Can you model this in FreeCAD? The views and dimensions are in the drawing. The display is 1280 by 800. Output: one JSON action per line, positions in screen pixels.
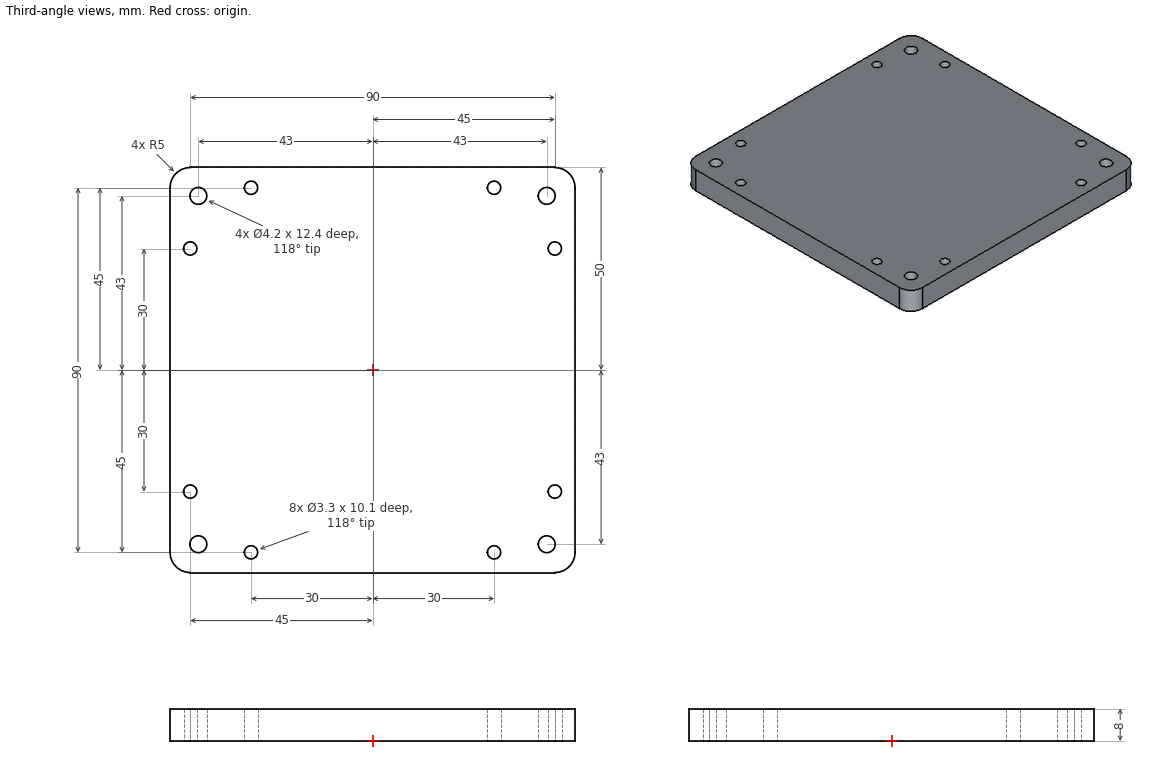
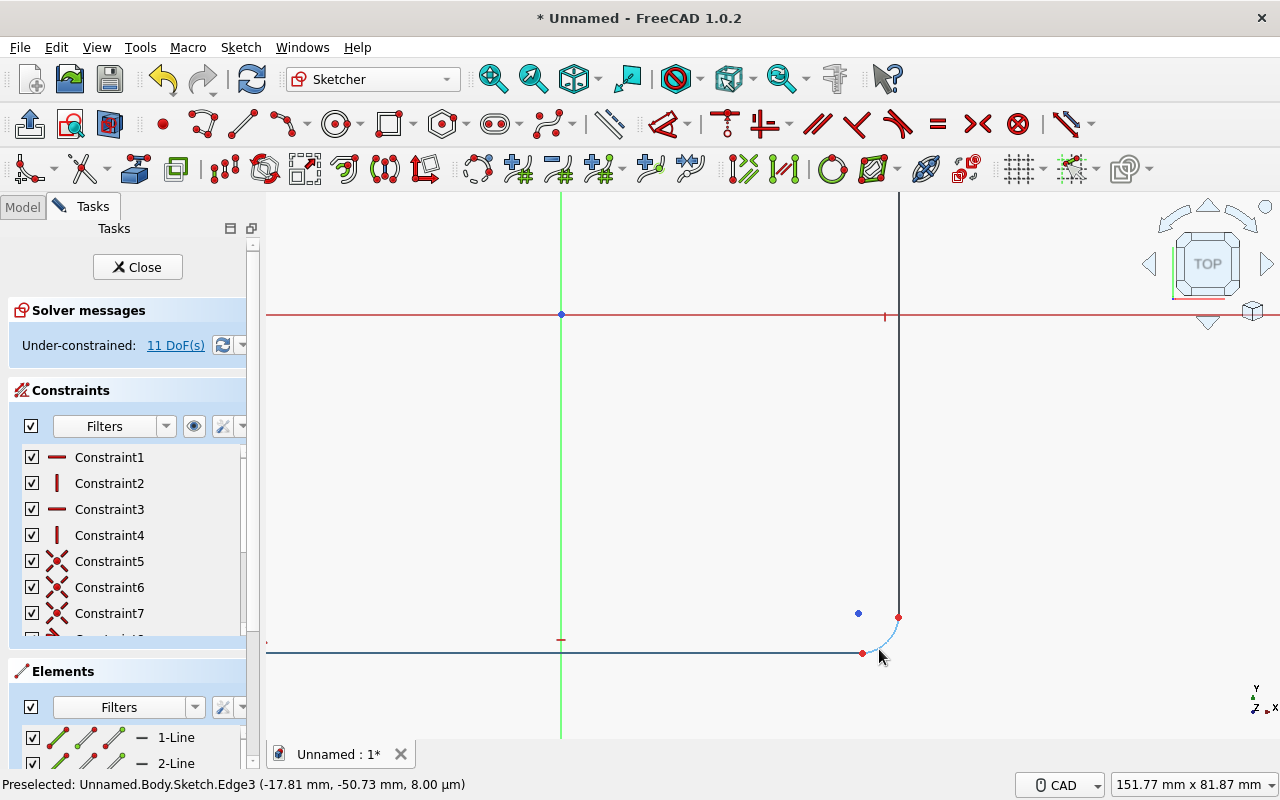
{"action": "left_click", "coordinate": [878, 649]}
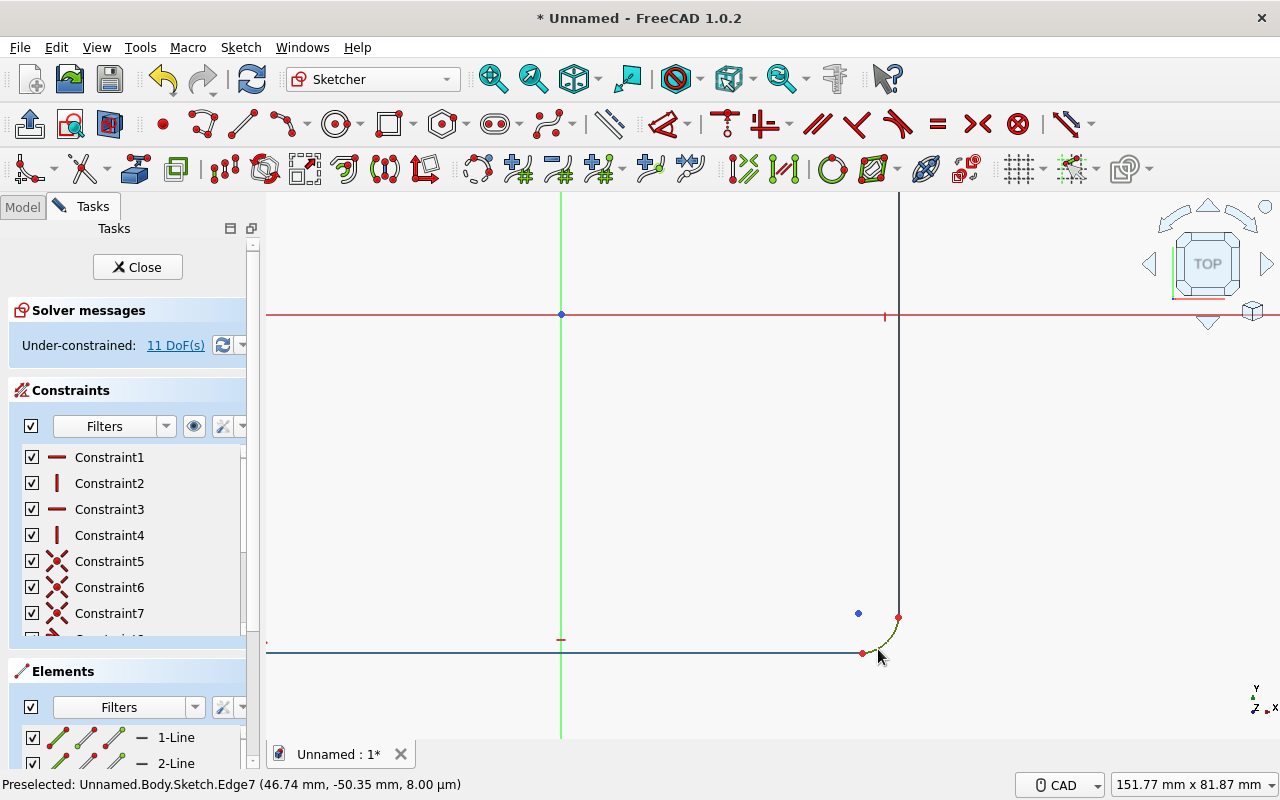
{"action": "left_click", "coordinate": [898, 124]}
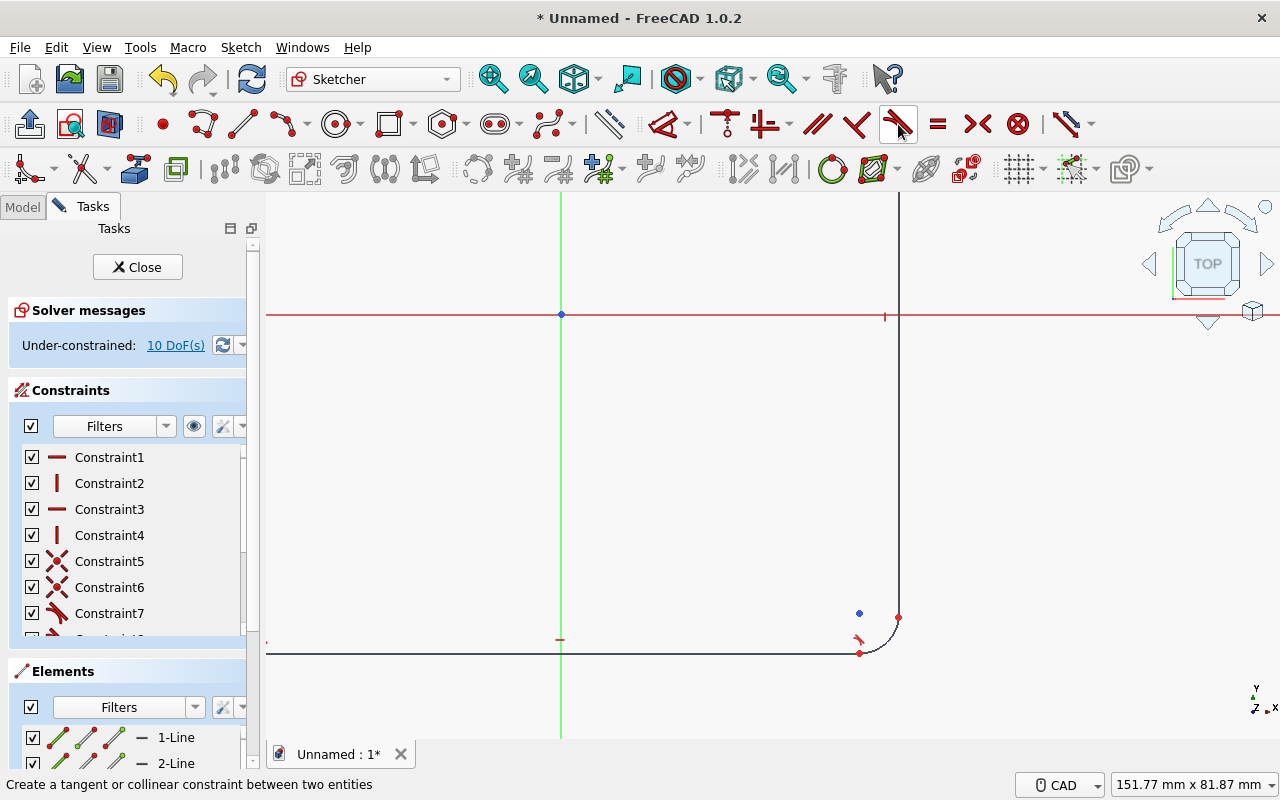
{"action": "left_click", "coordinate": [899, 437]}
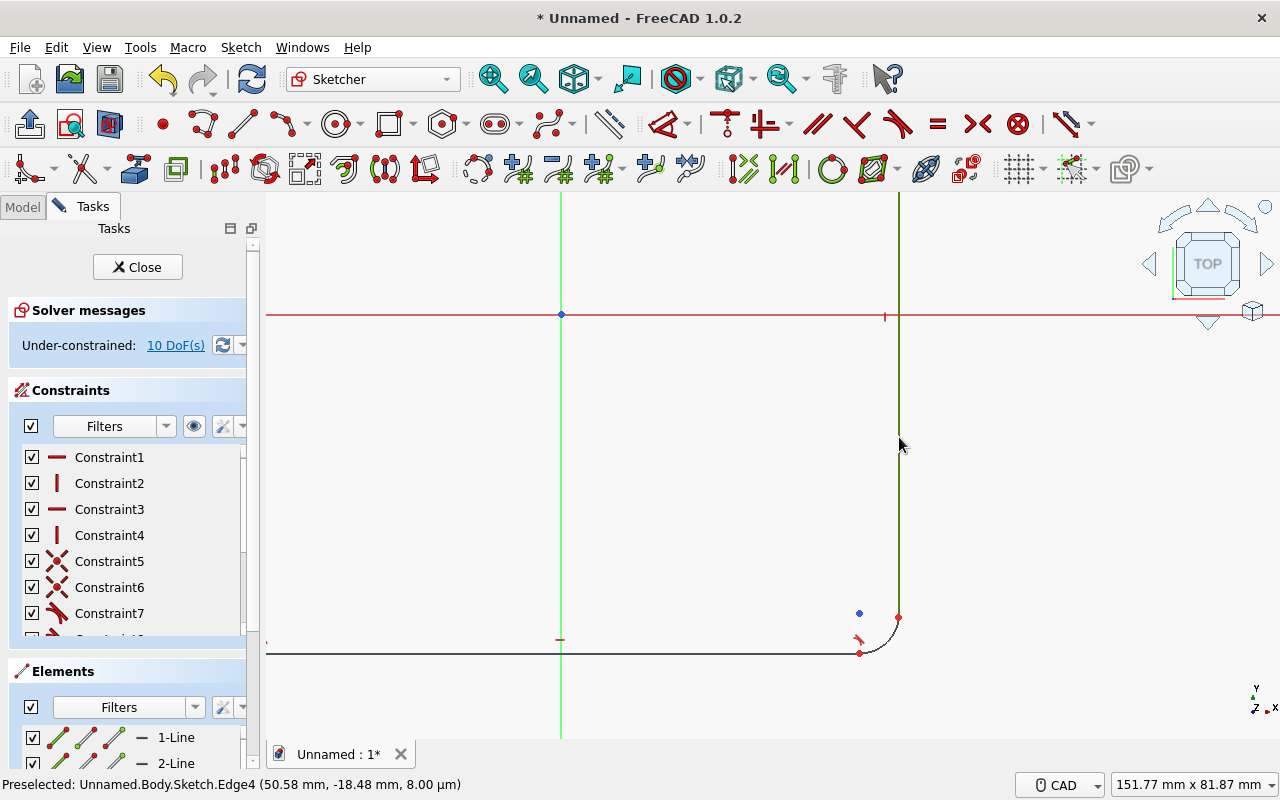
{"action": "left_click", "coordinate": [876, 650]}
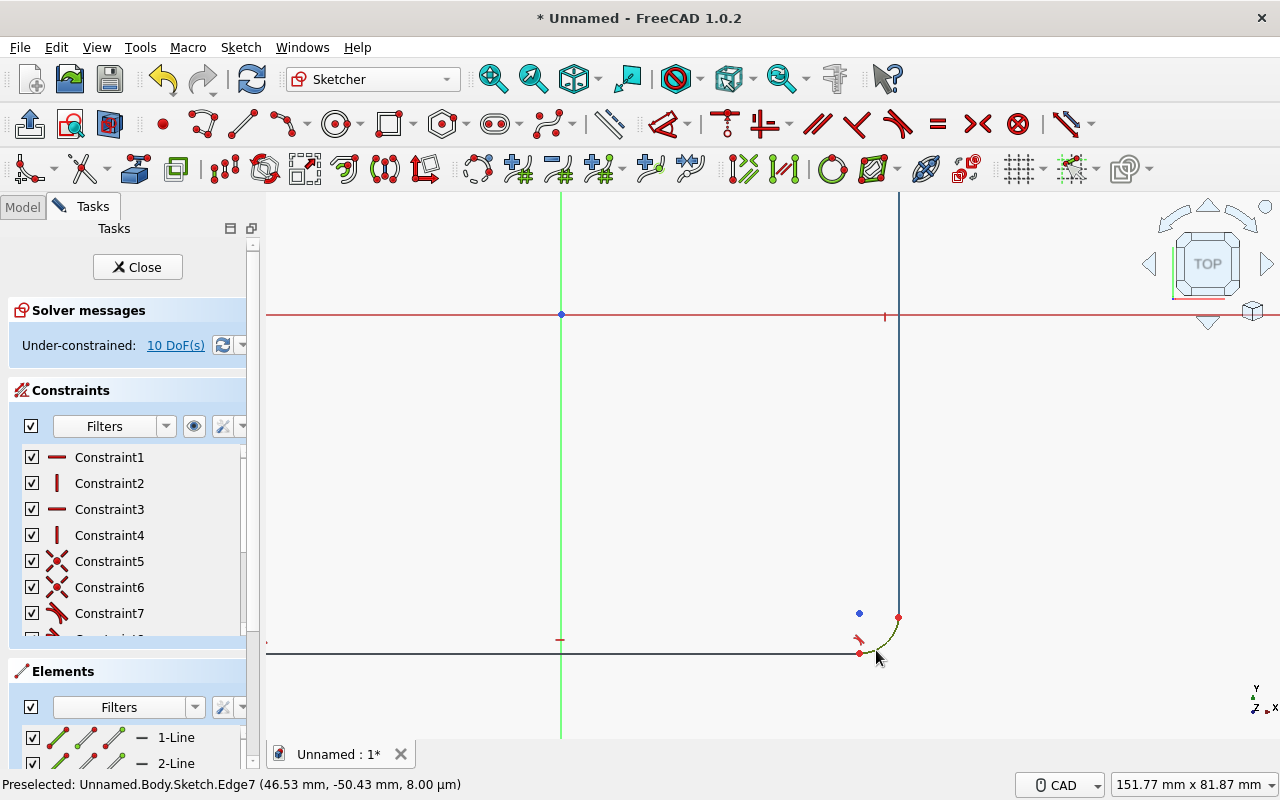
{"action": "key", "text": "t"}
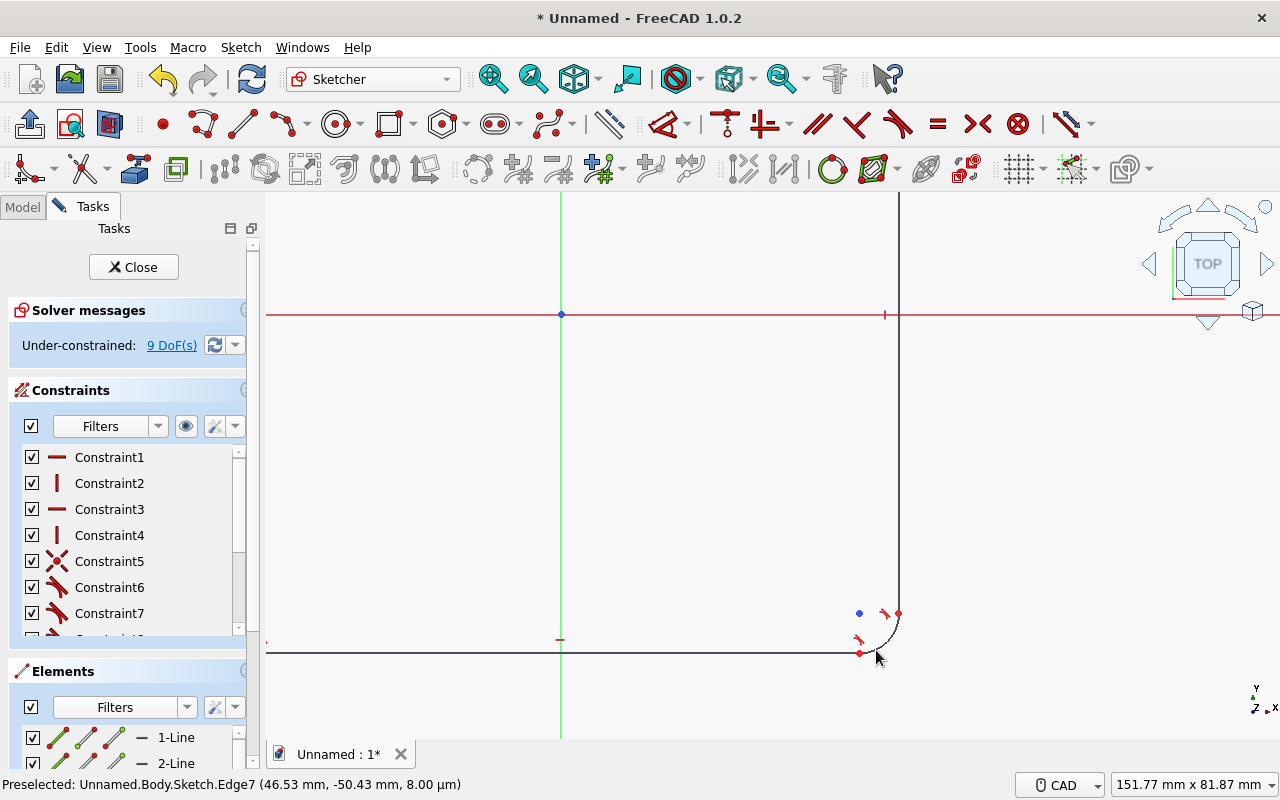
{"action": "left_click", "coordinate": [899, 434]}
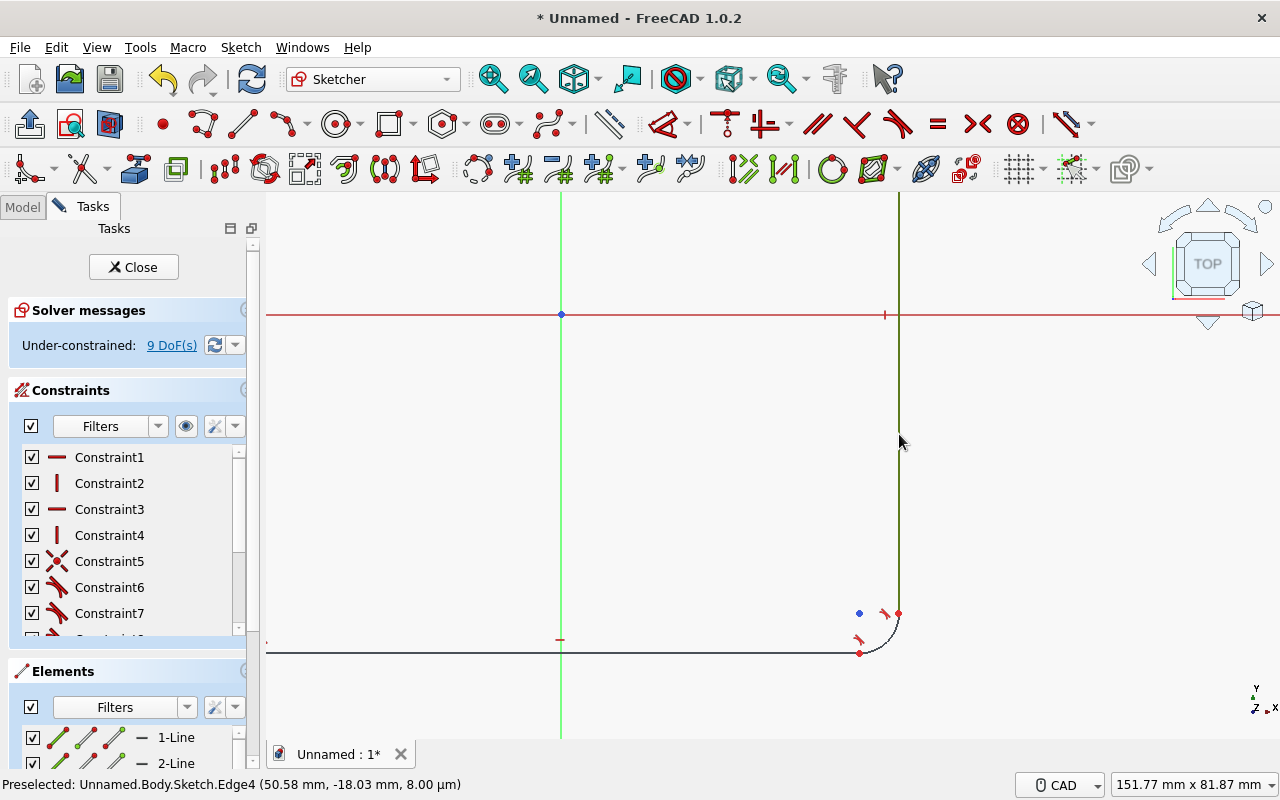
{"action": "scroll", "coordinate": [879, 649], "scroll_direction": "down", "scroll_amount": 3}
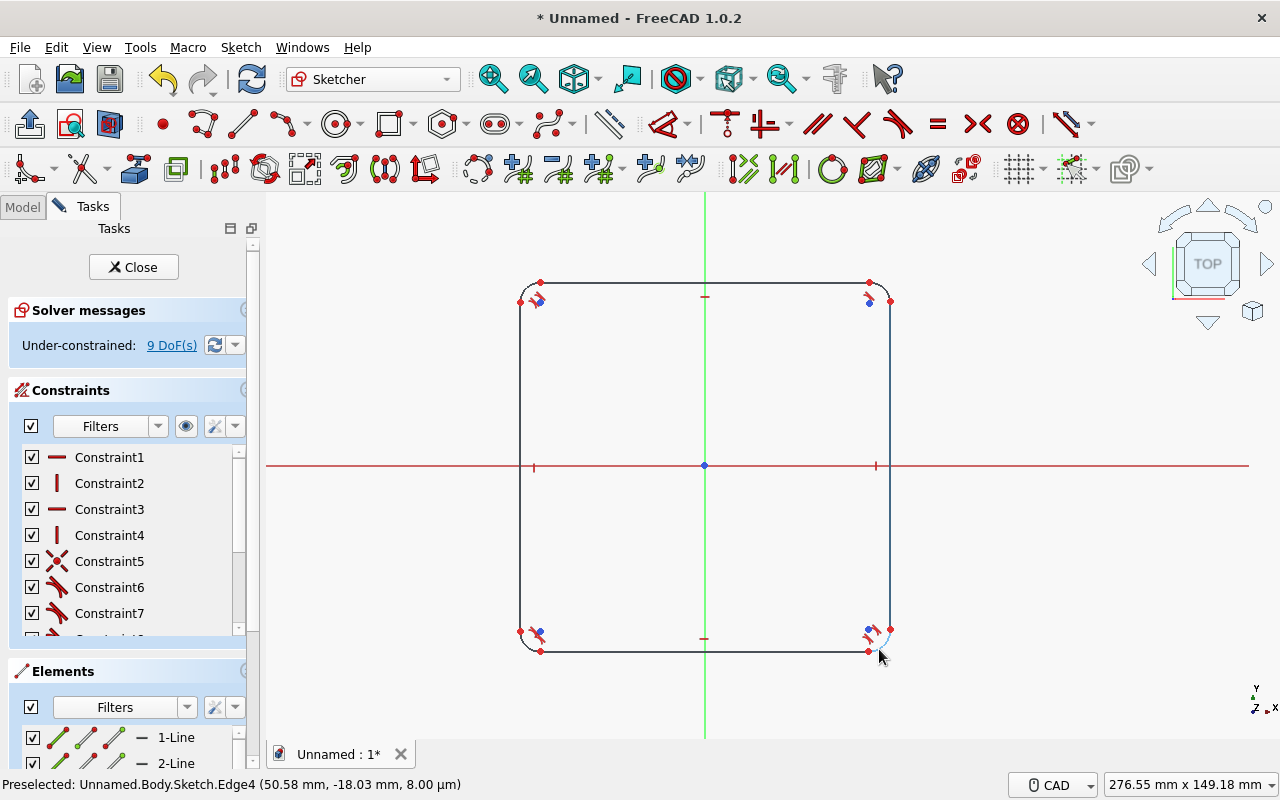
{"action": "scroll", "coordinate": [888, 293], "scroll_direction": "up", "scroll_amount": 3}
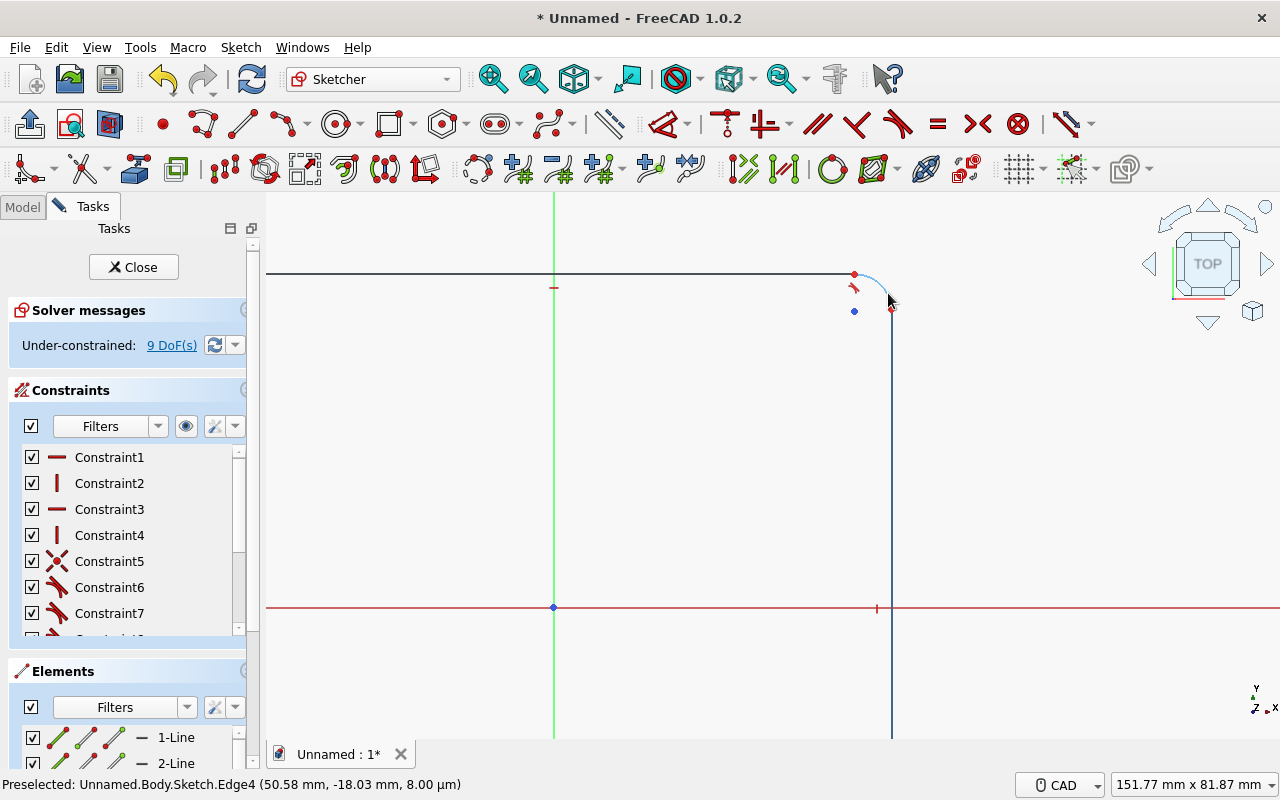
{"action": "left_click", "coordinate": [887, 293]}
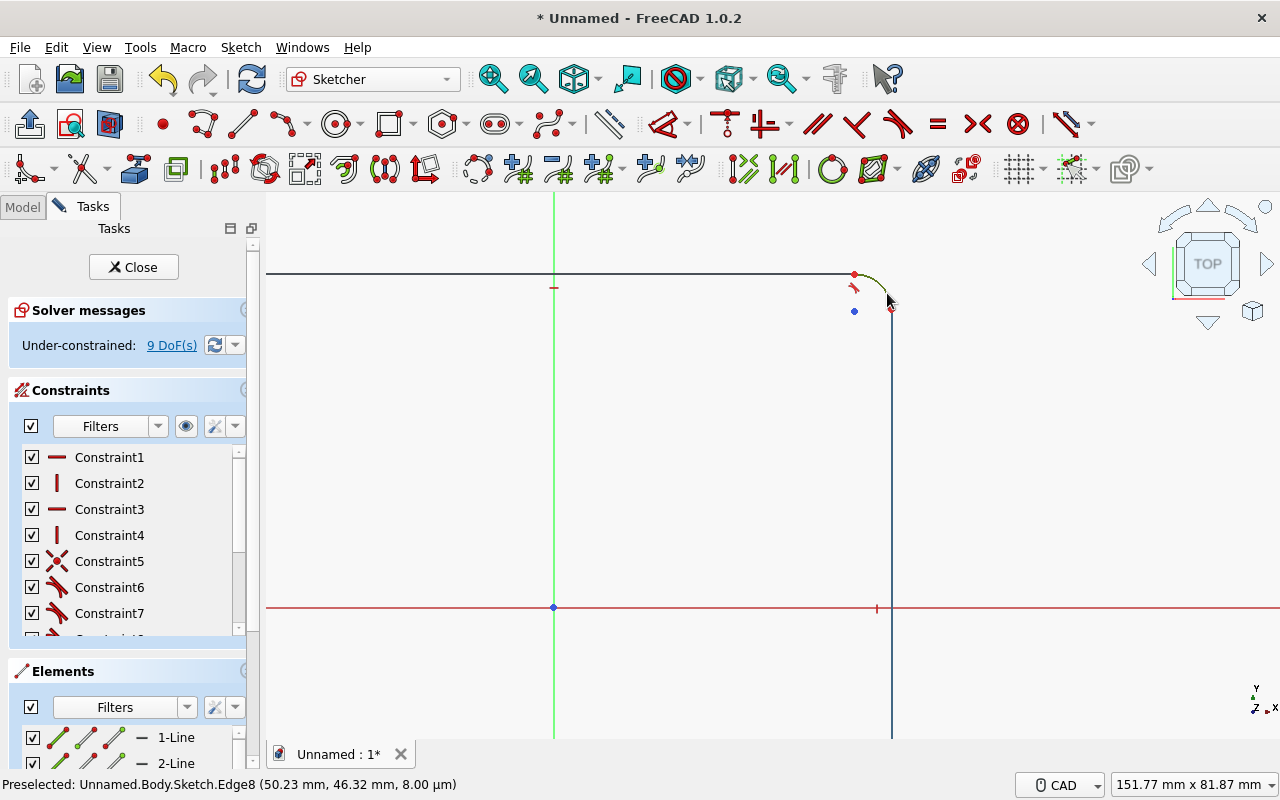
{"action": "key", "text": "t"}